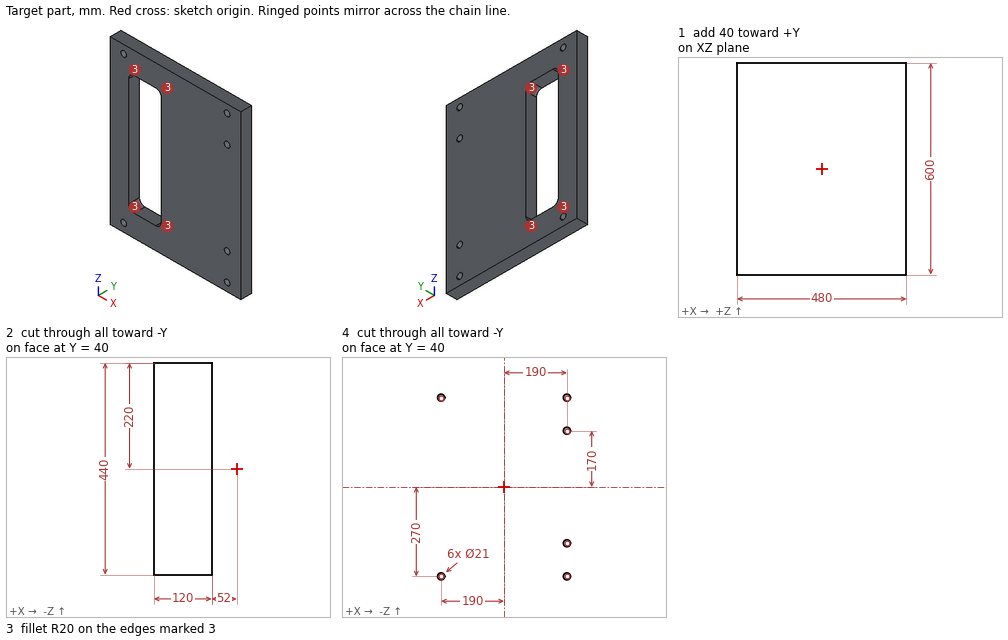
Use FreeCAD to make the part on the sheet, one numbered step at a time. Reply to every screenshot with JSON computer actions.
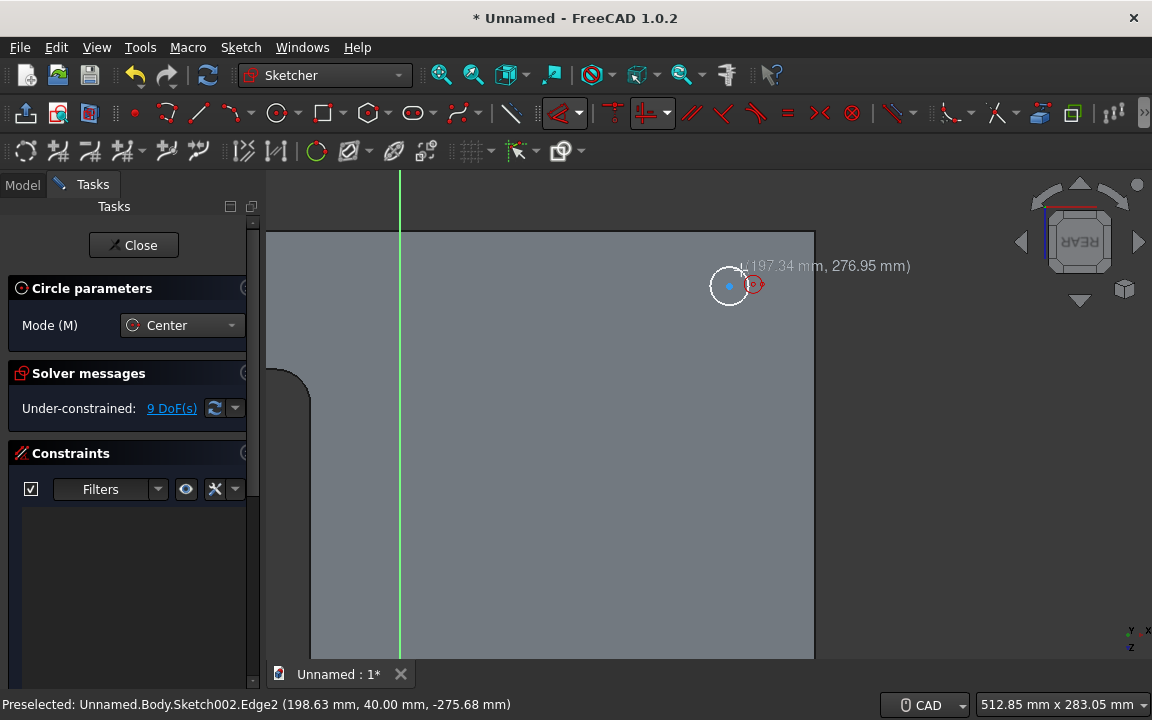
{"action": "scroll", "coordinate": [744, 270], "scroll_direction": "down", "scroll_amount": 6}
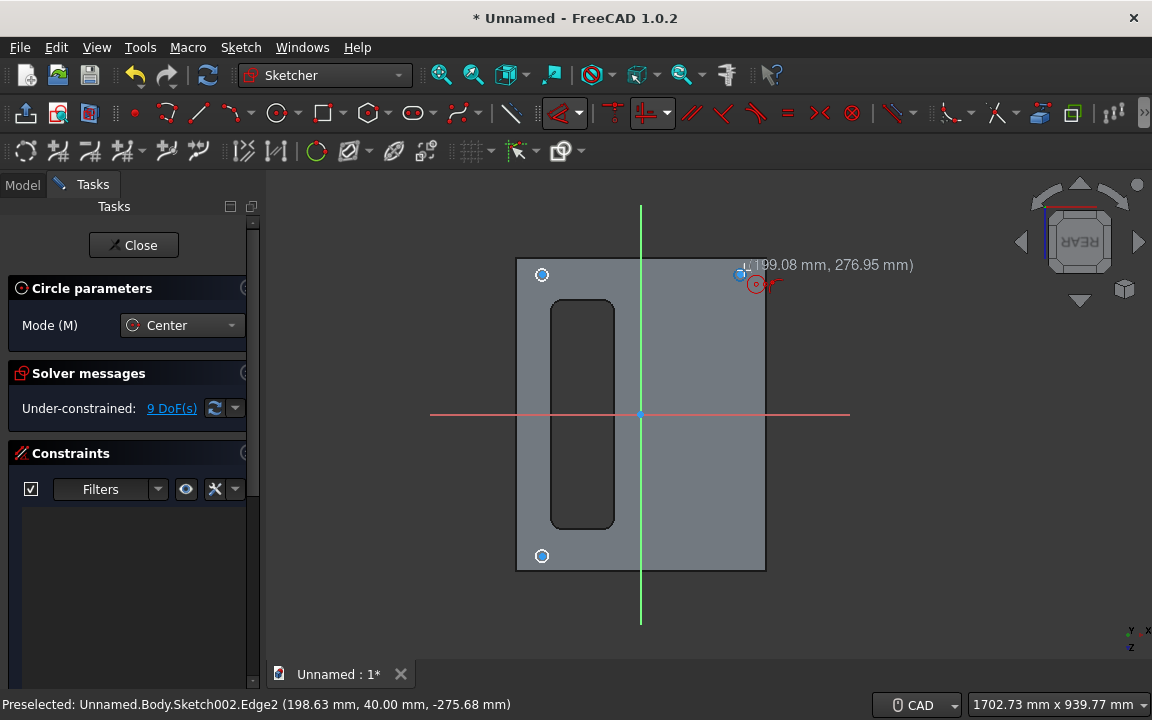
{"action": "scroll", "coordinate": [740, 555], "scroll_direction": "up", "scroll_amount": 8}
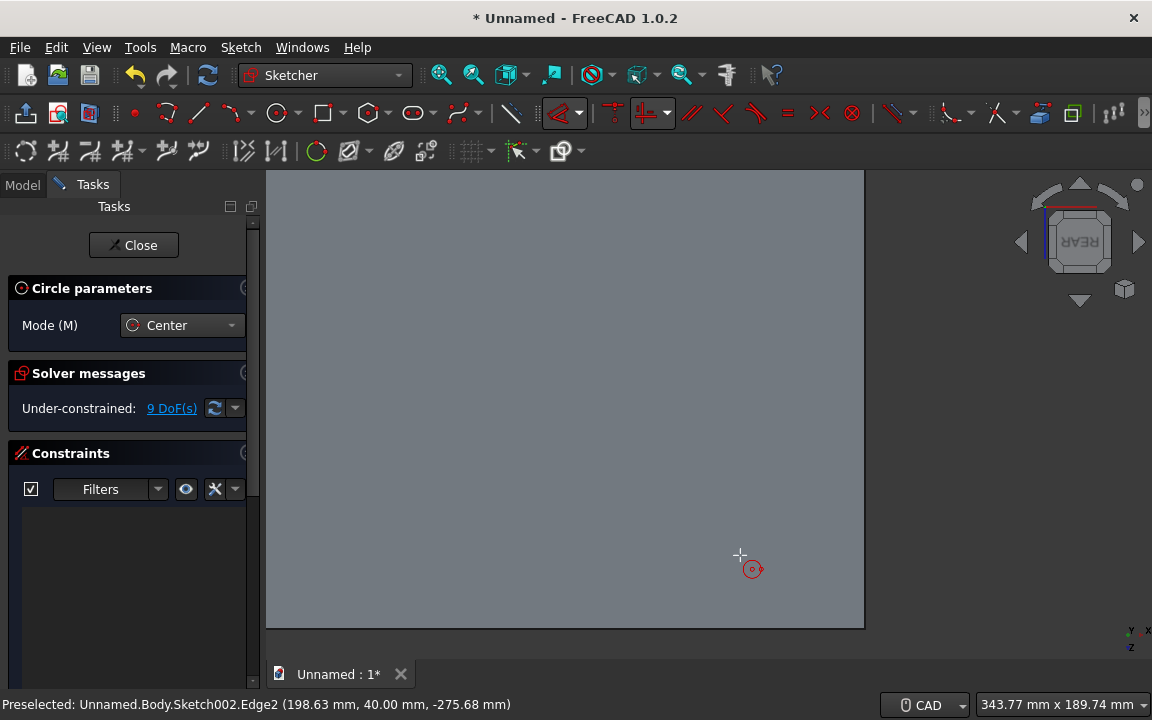
{"action": "scroll", "coordinate": [740, 556], "scroll_direction": "down", "scroll_amount": 8}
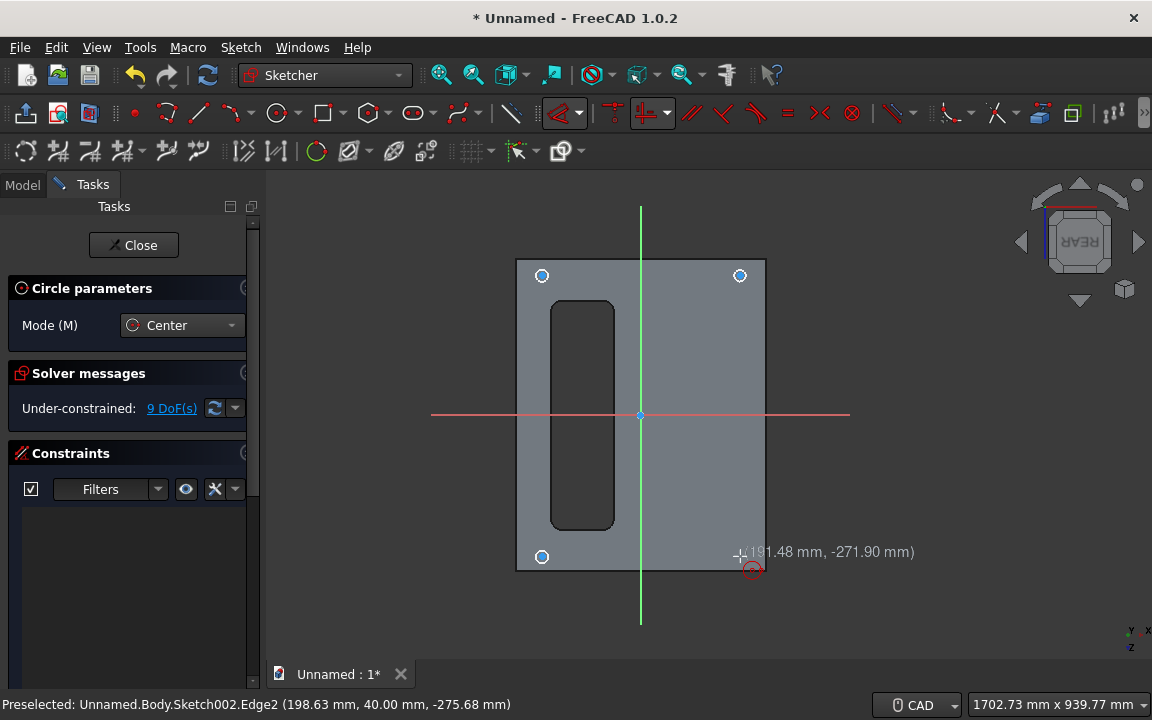
{"action": "left_click", "coordinate": [740, 556]}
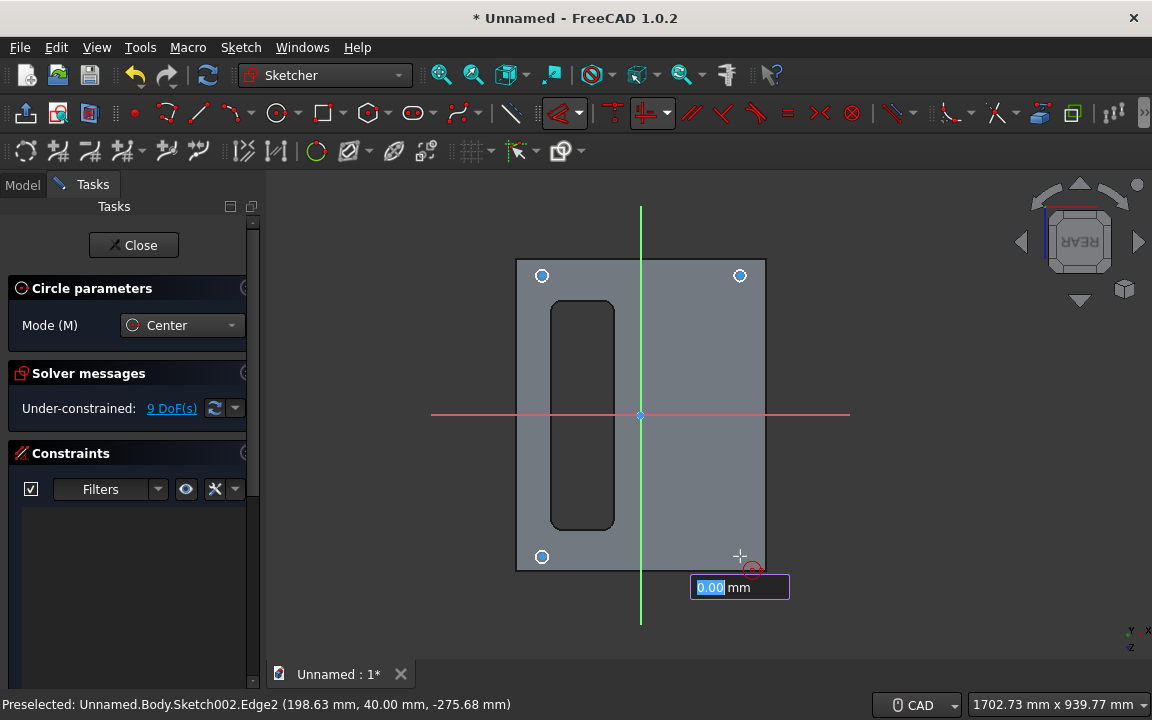
{"action": "scroll", "coordinate": [744, 552], "scroll_direction": "up", "scroll_amount": 6}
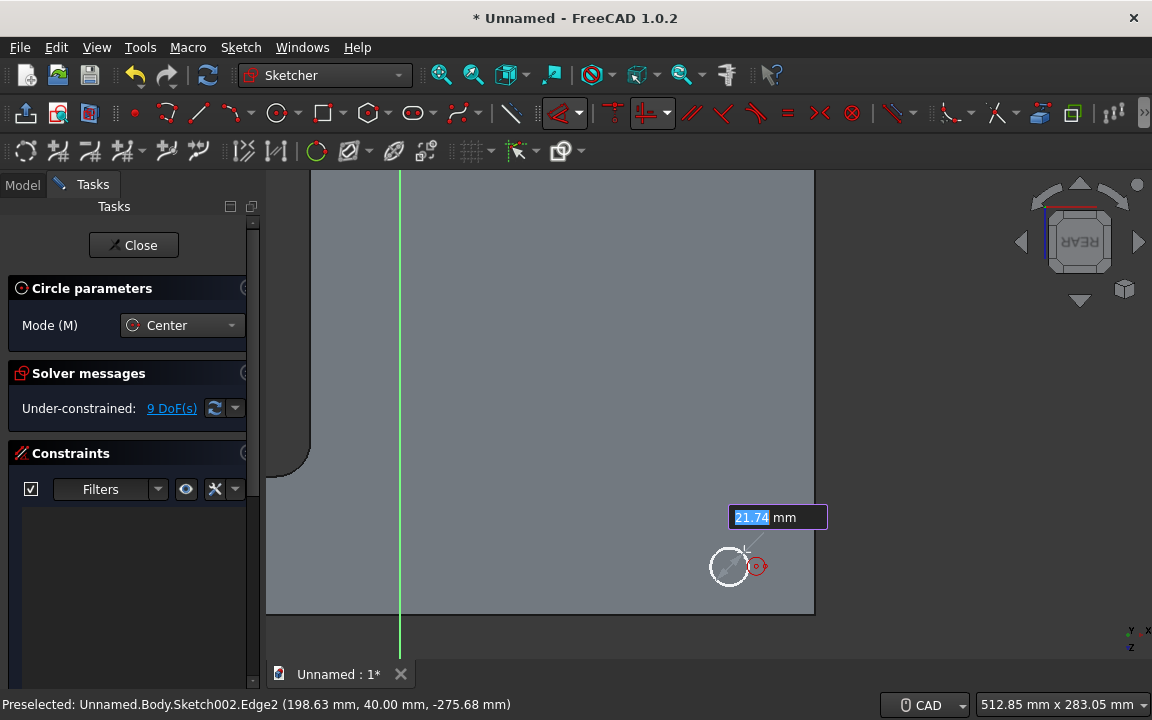
{"action": "left_click", "coordinate": [741, 550]}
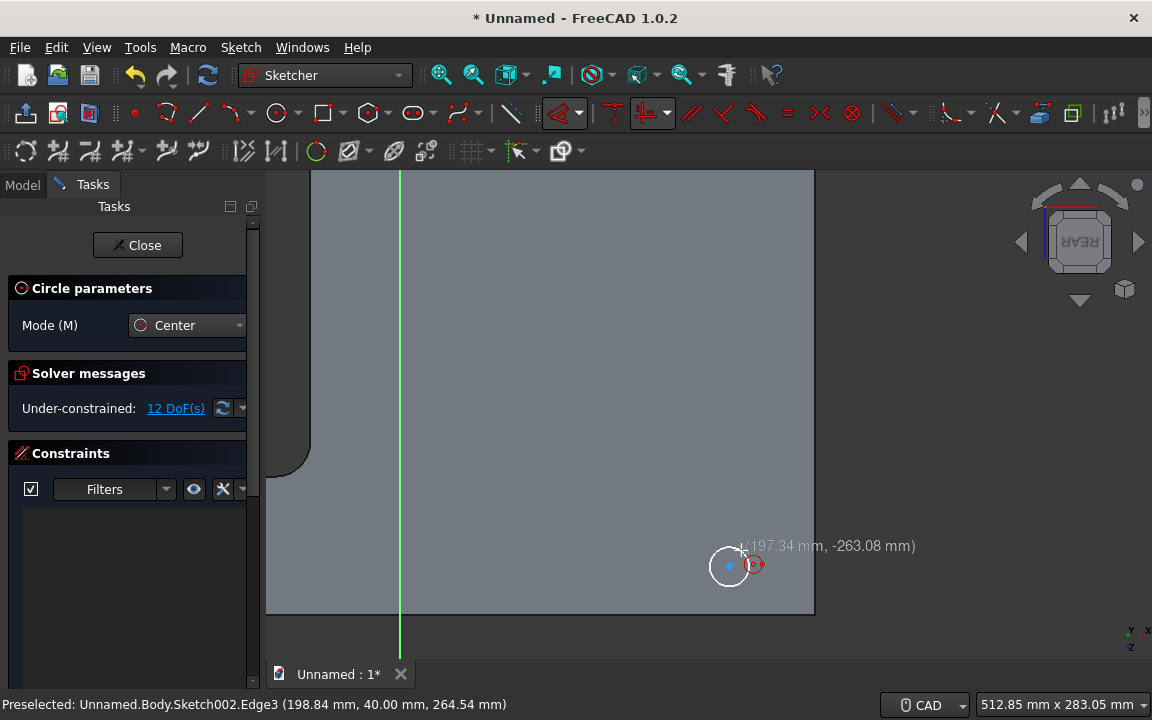
{"action": "scroll", "coordinate": [744, 552], "scroll_direction": "down", "scroll_amount": 6}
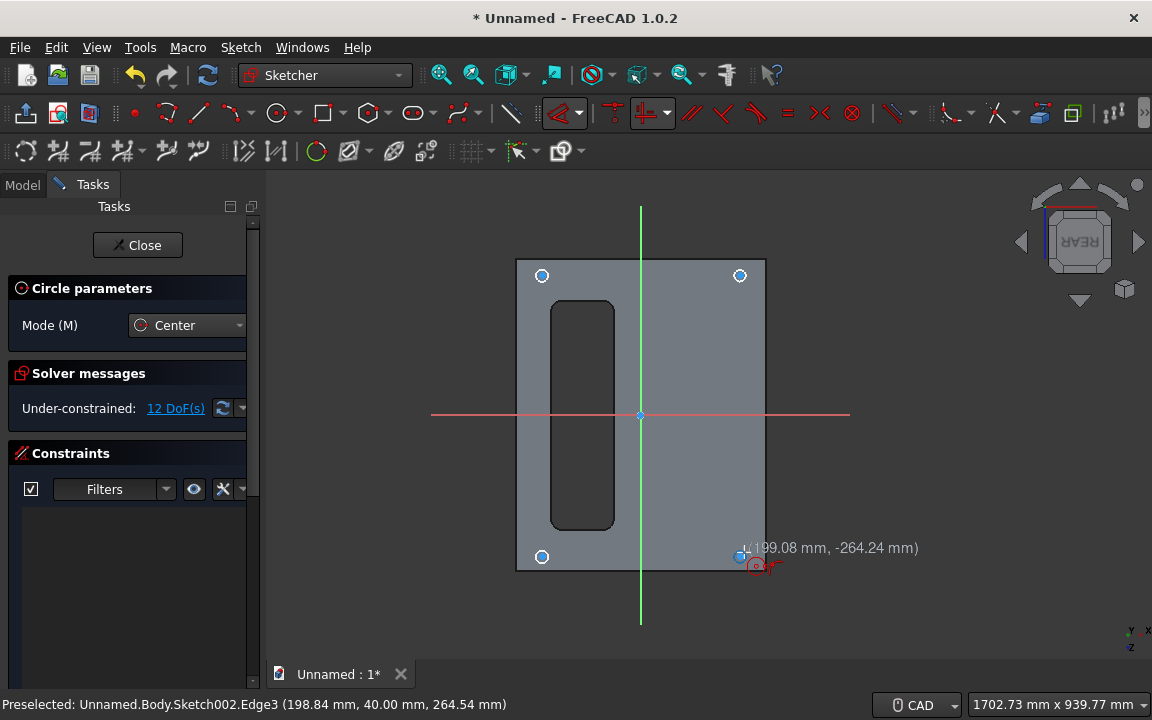
{"action": "scroll", "coordinate": [740, 327], "scroll_direction": "up", "scroll_amount": 8}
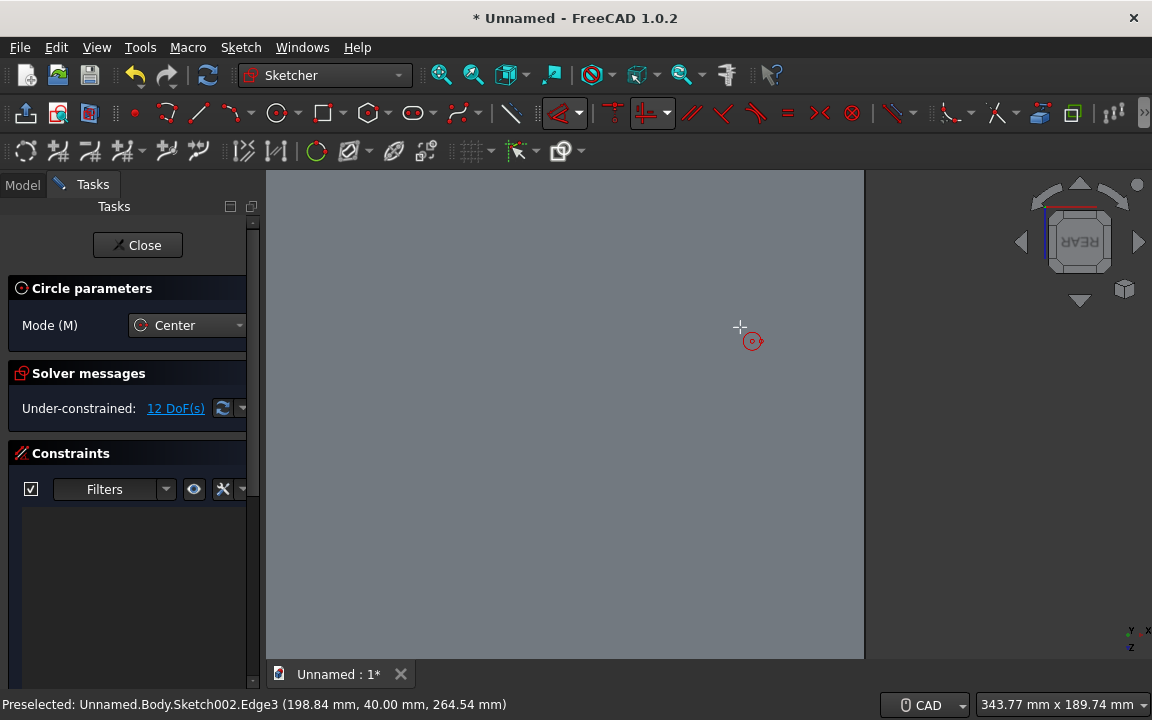
{"action": "scroll", "coordinate": [740, 326], "scroll_direction": "down", "scroll_amount": 8}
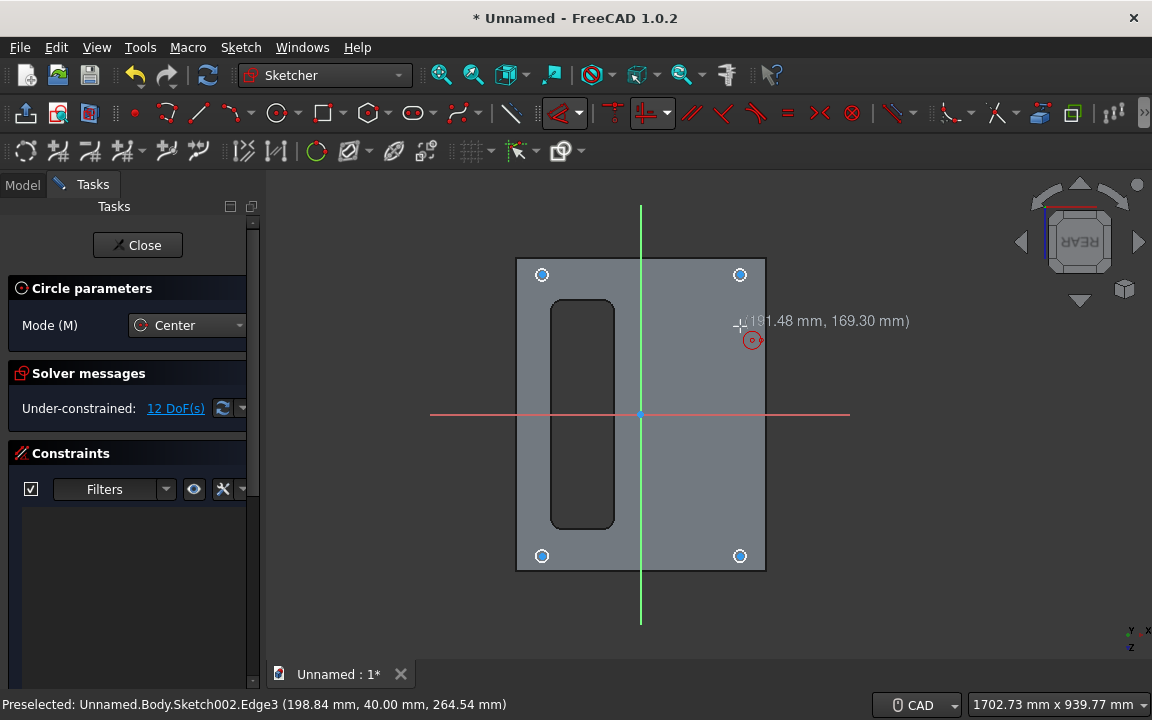
{"action": "left_click", "coordinate": [740, 326]}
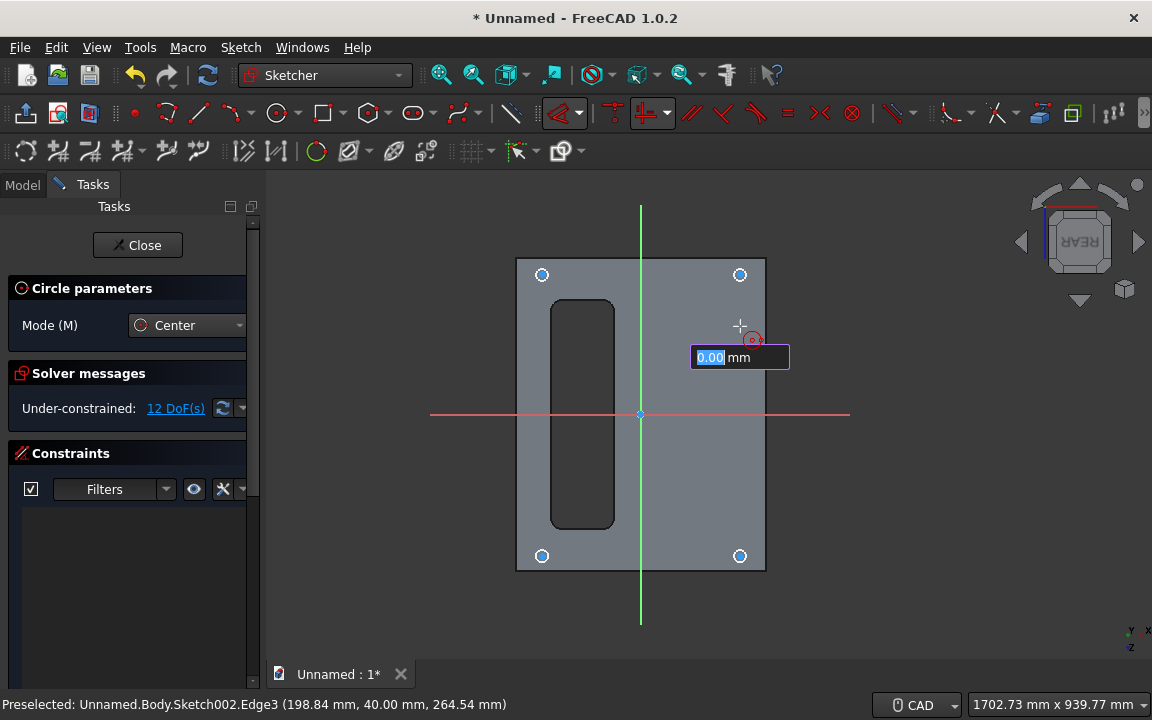
{"action": "scroll", "coordinate": [744, 322], "scroll_direction": "up", "scroll_amount": 6}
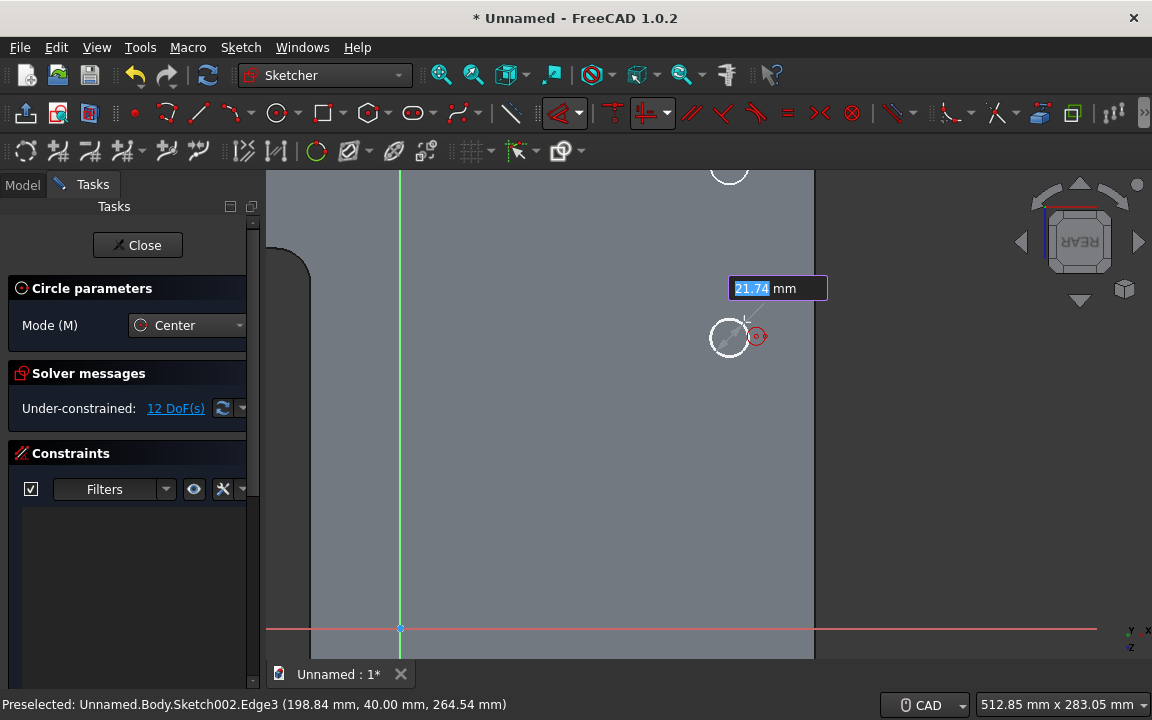
{"action": "left_click", "coordinate": [741, 322]}